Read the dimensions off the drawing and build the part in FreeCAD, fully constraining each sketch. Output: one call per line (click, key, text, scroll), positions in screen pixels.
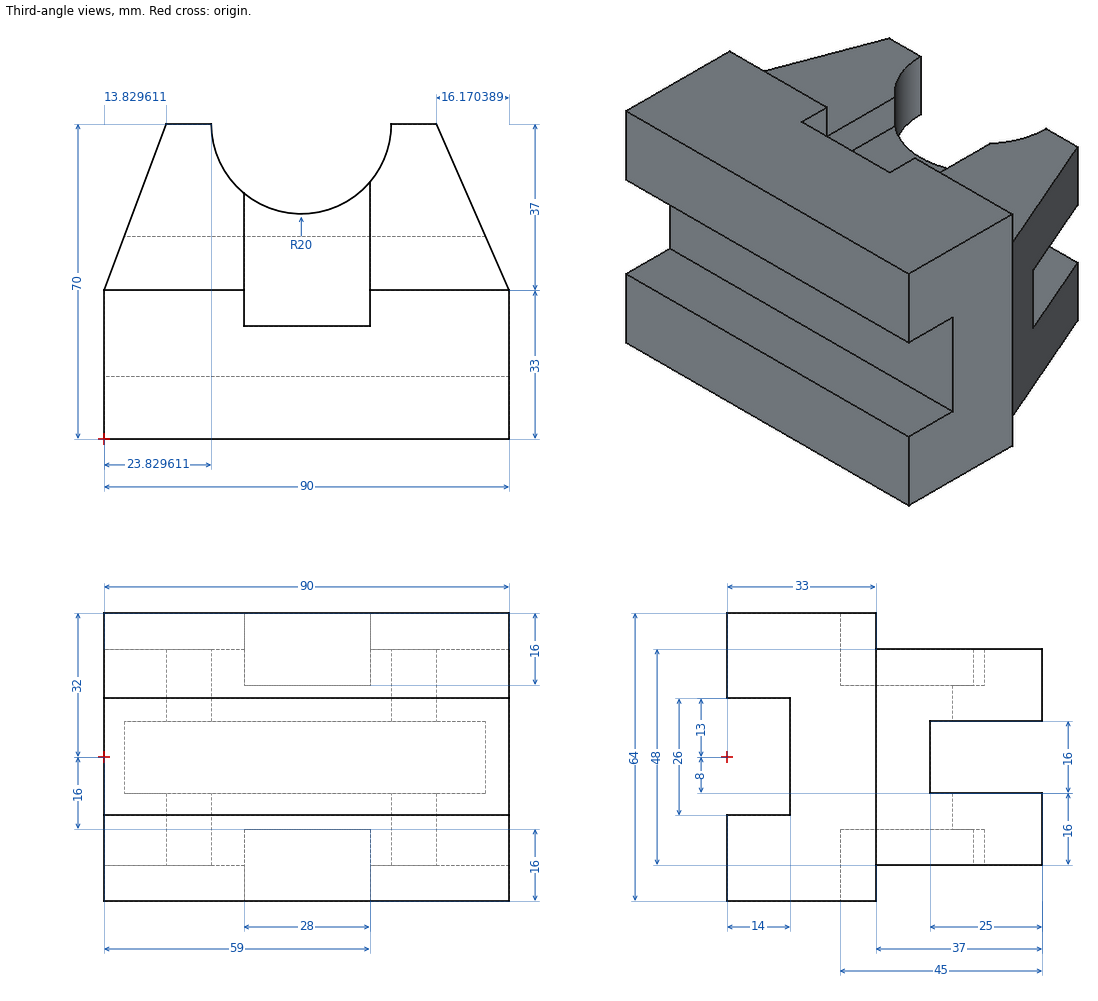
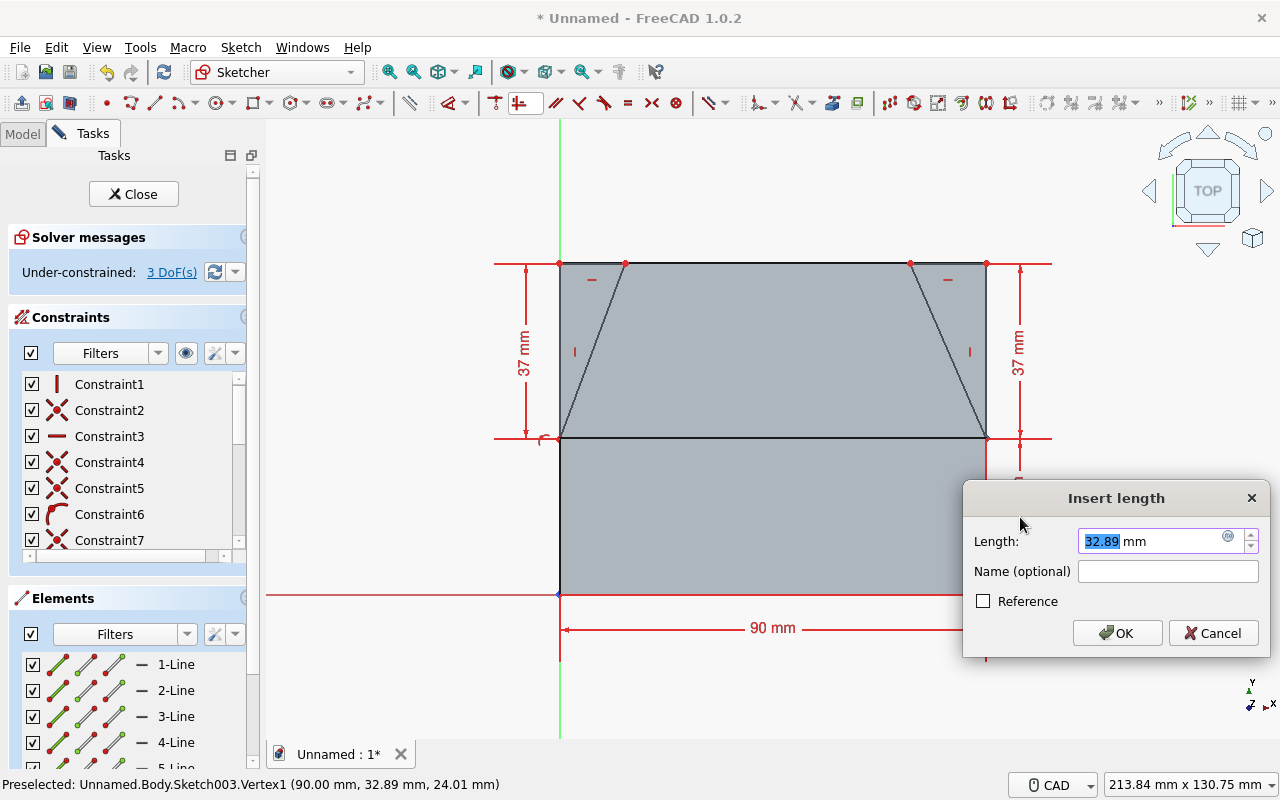
text(33)
key(Return)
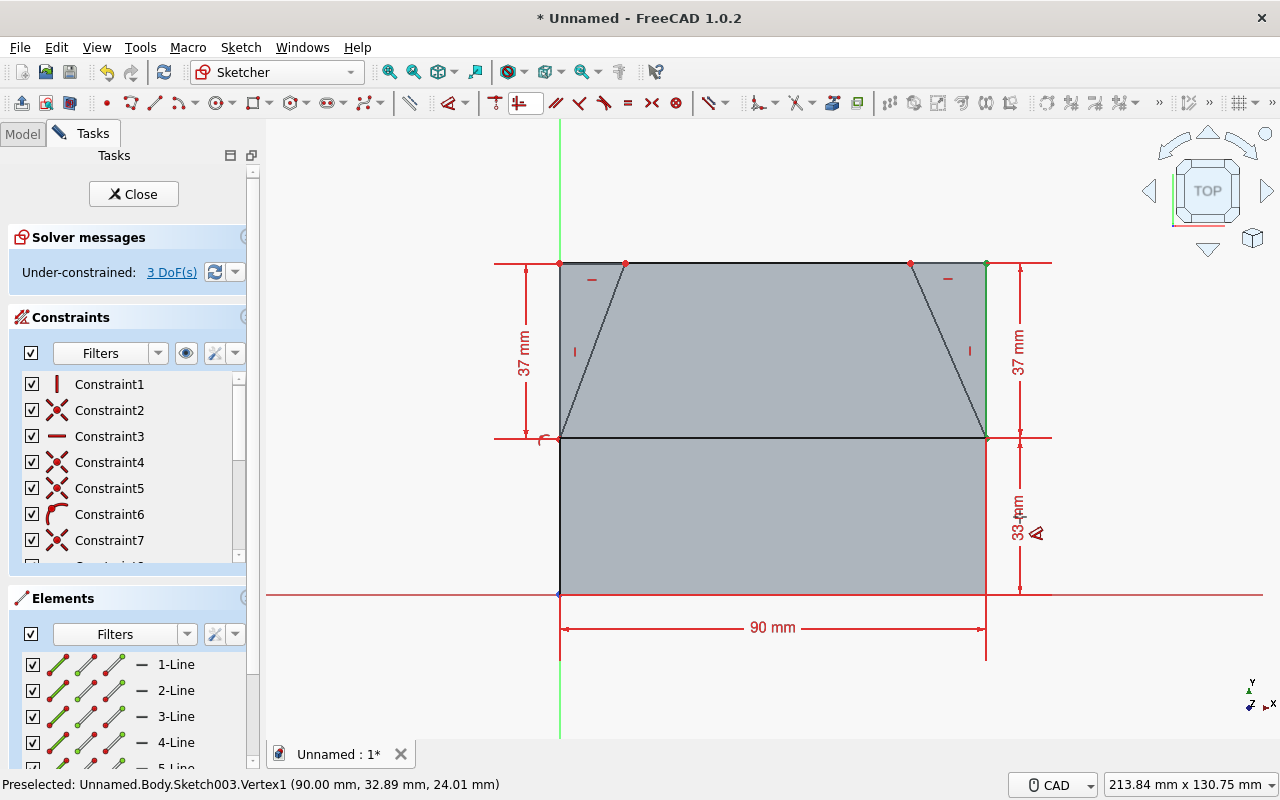
click(560, 439)
click(526, 517)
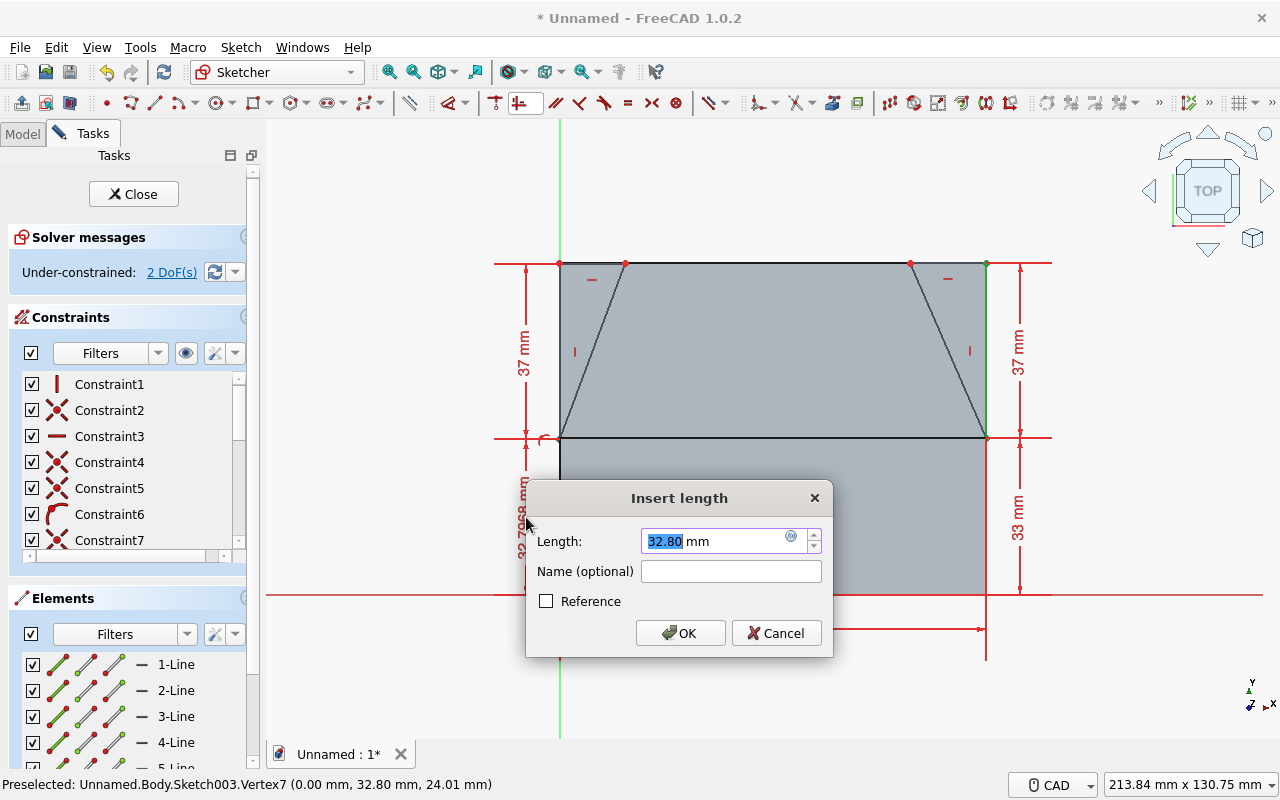
text(33)
key(Return)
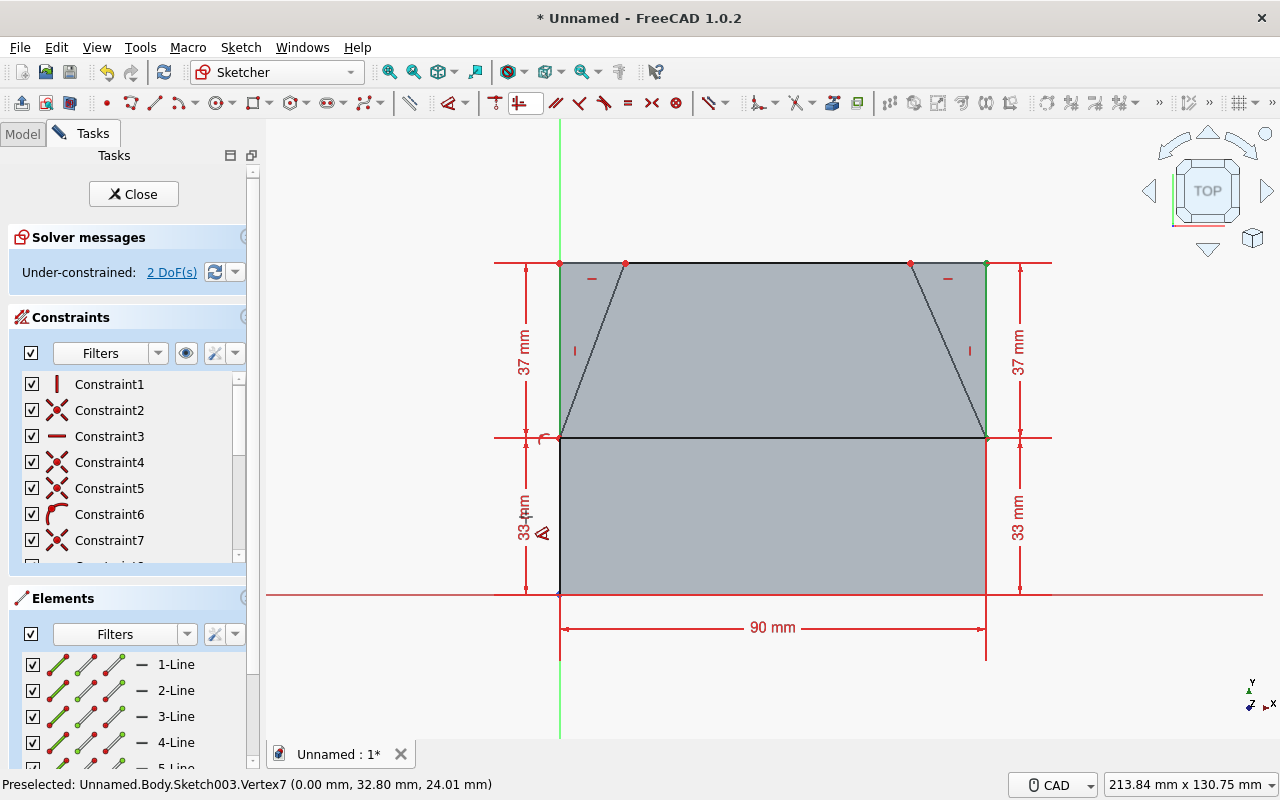
click(963, 263)
click(948, 229)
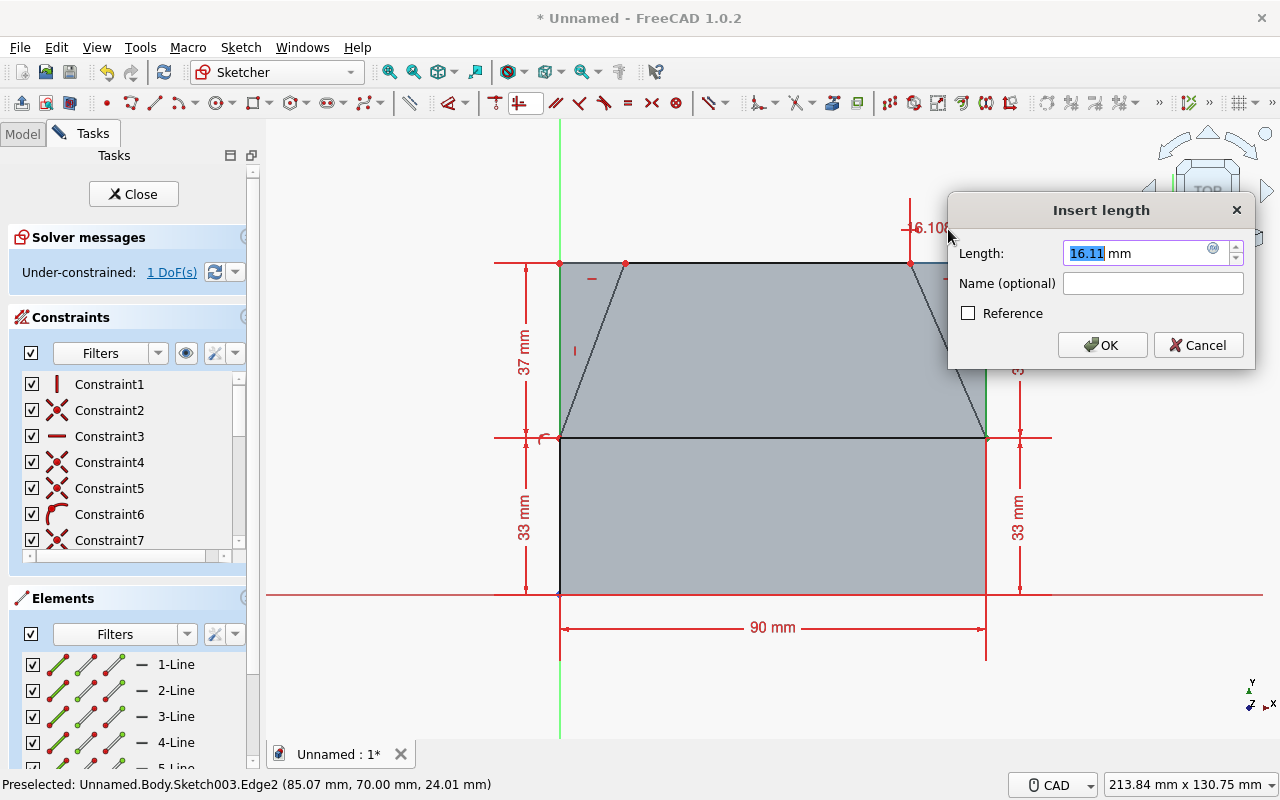
text(16.170389)
key(Return)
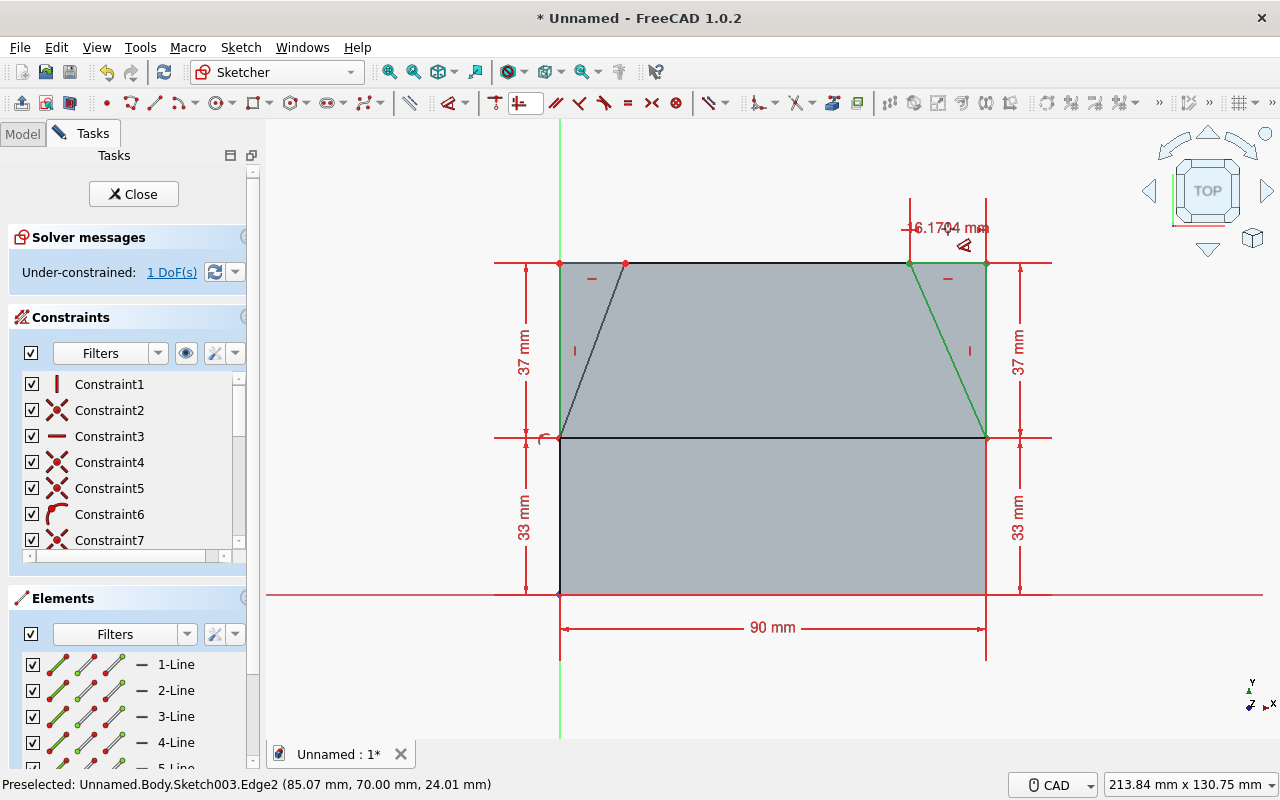
click(605, 263)
click(592, 229)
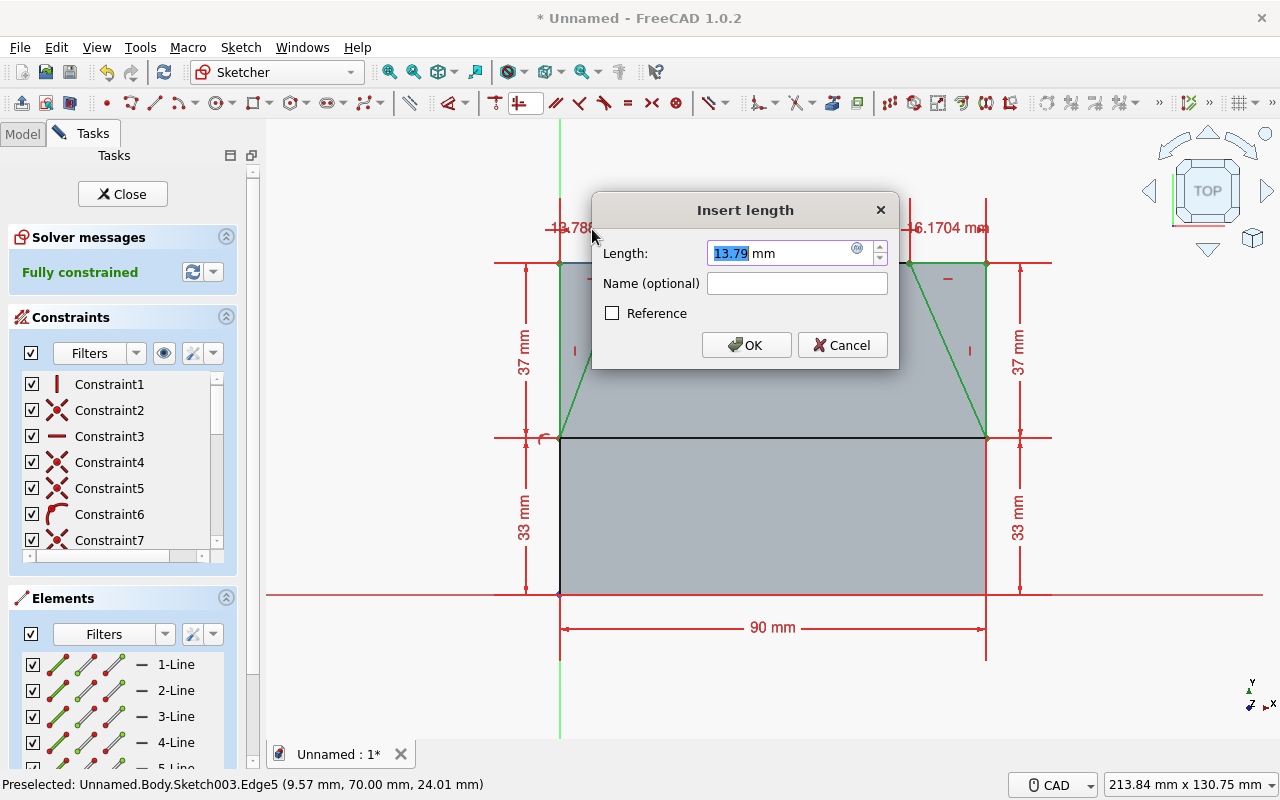
text(13.829611)
key(Return)
key(Escape)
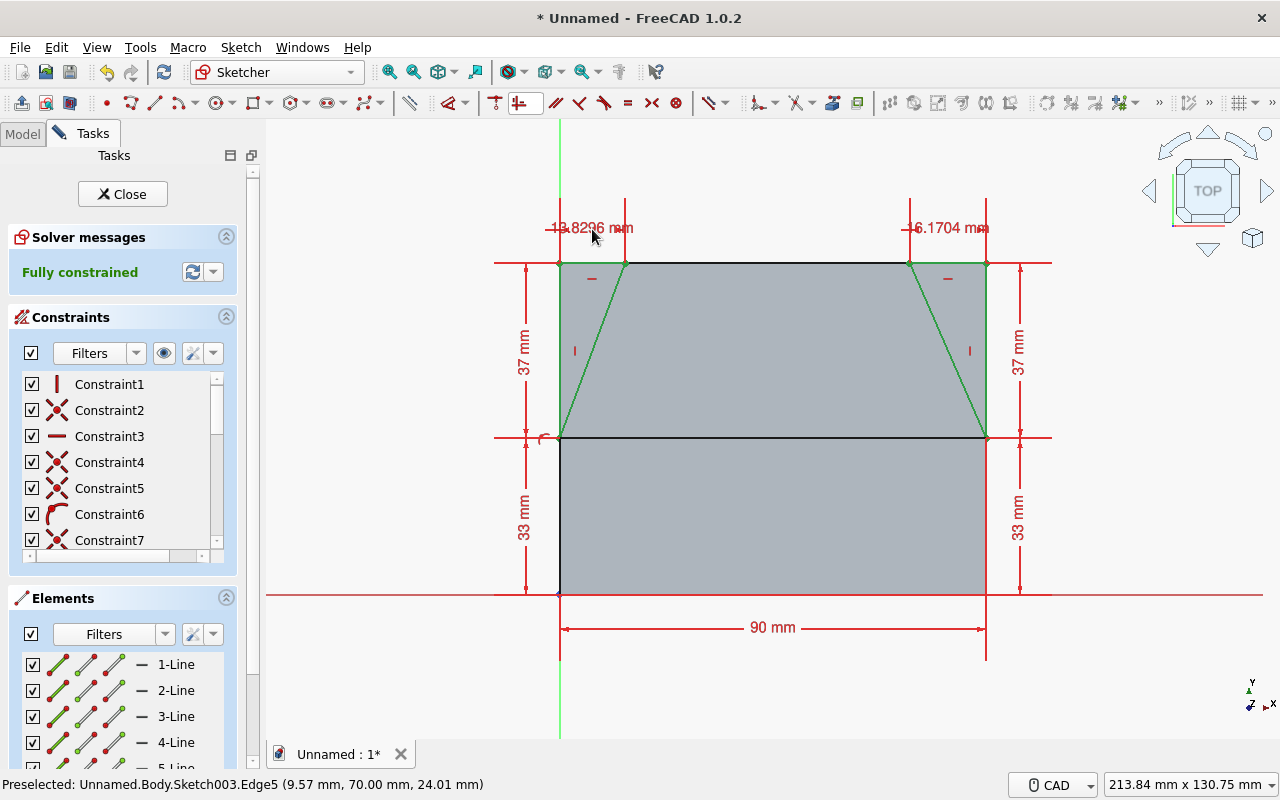
click(123, 194)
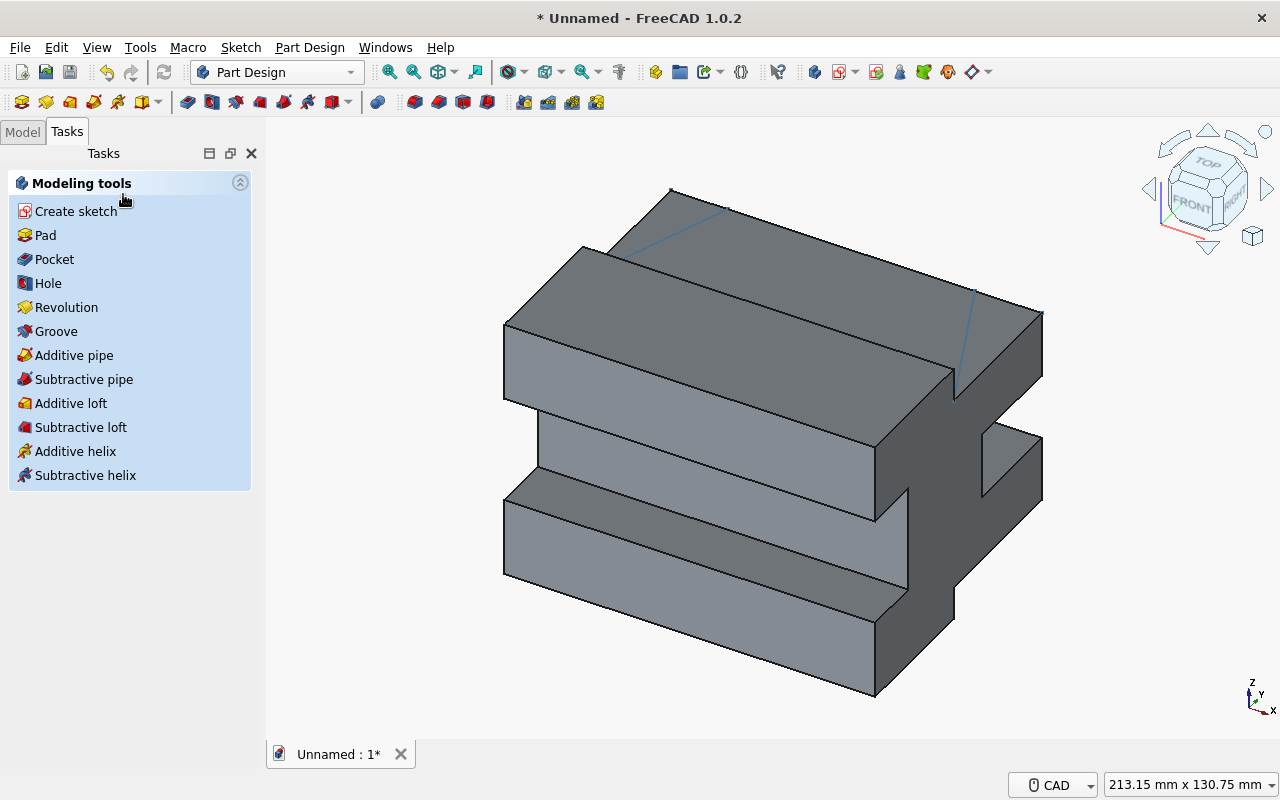
click(188, 102)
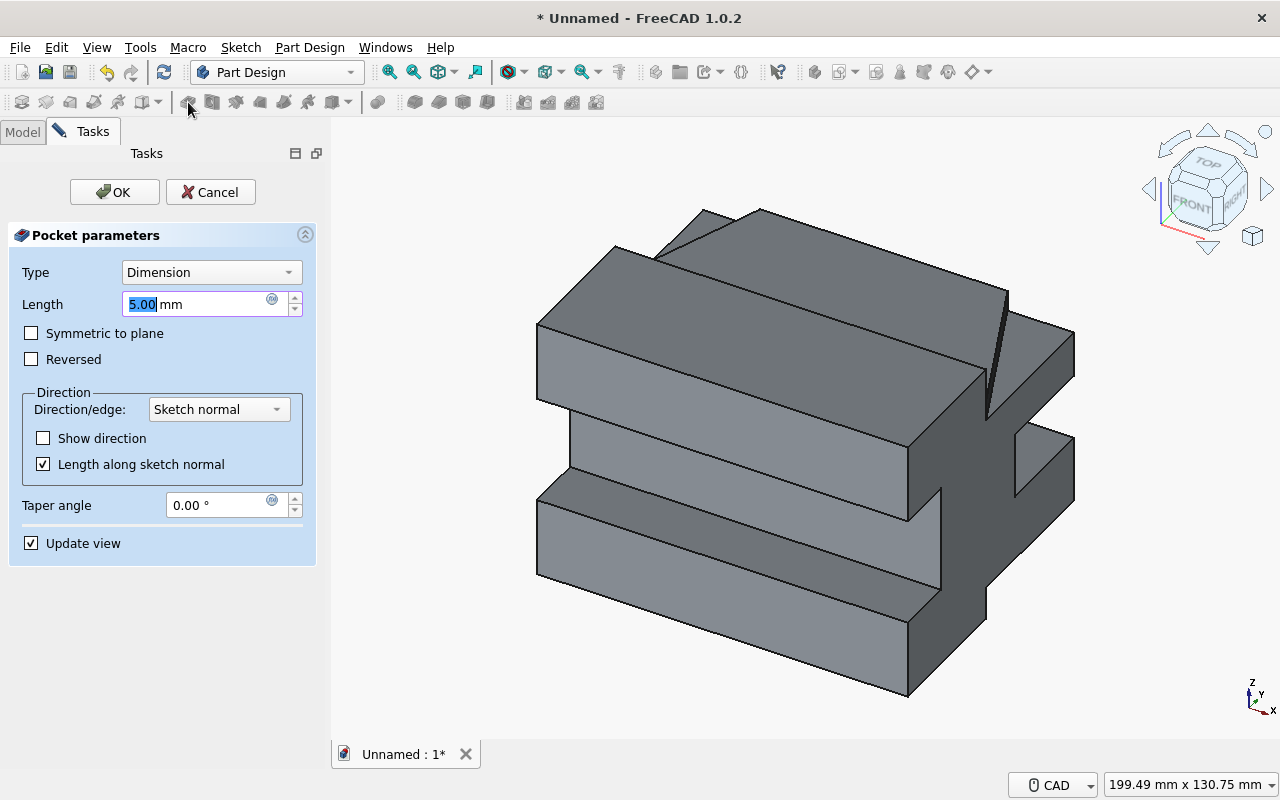
click(212, 272)